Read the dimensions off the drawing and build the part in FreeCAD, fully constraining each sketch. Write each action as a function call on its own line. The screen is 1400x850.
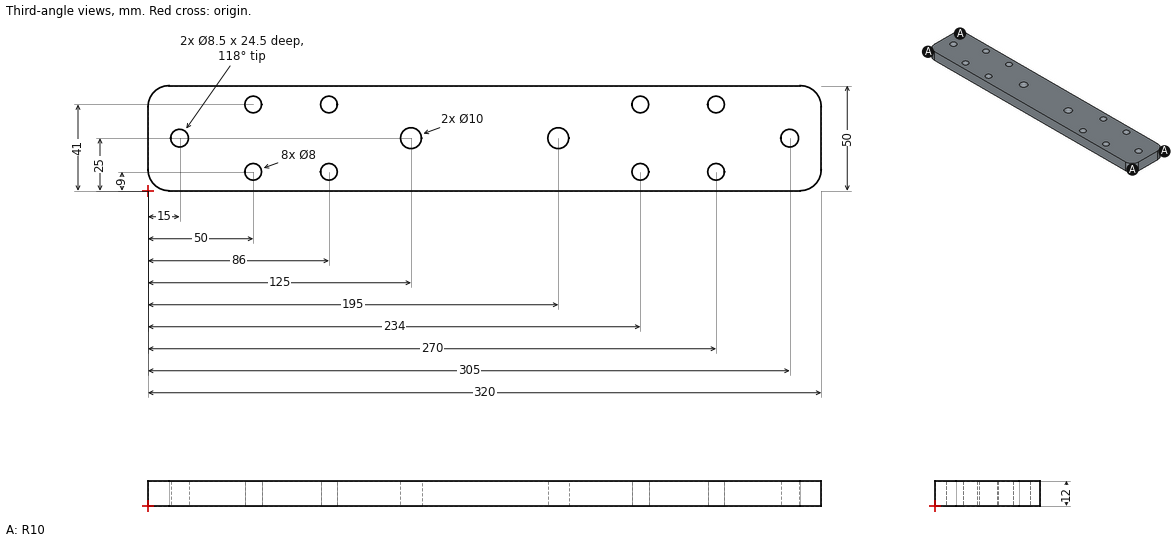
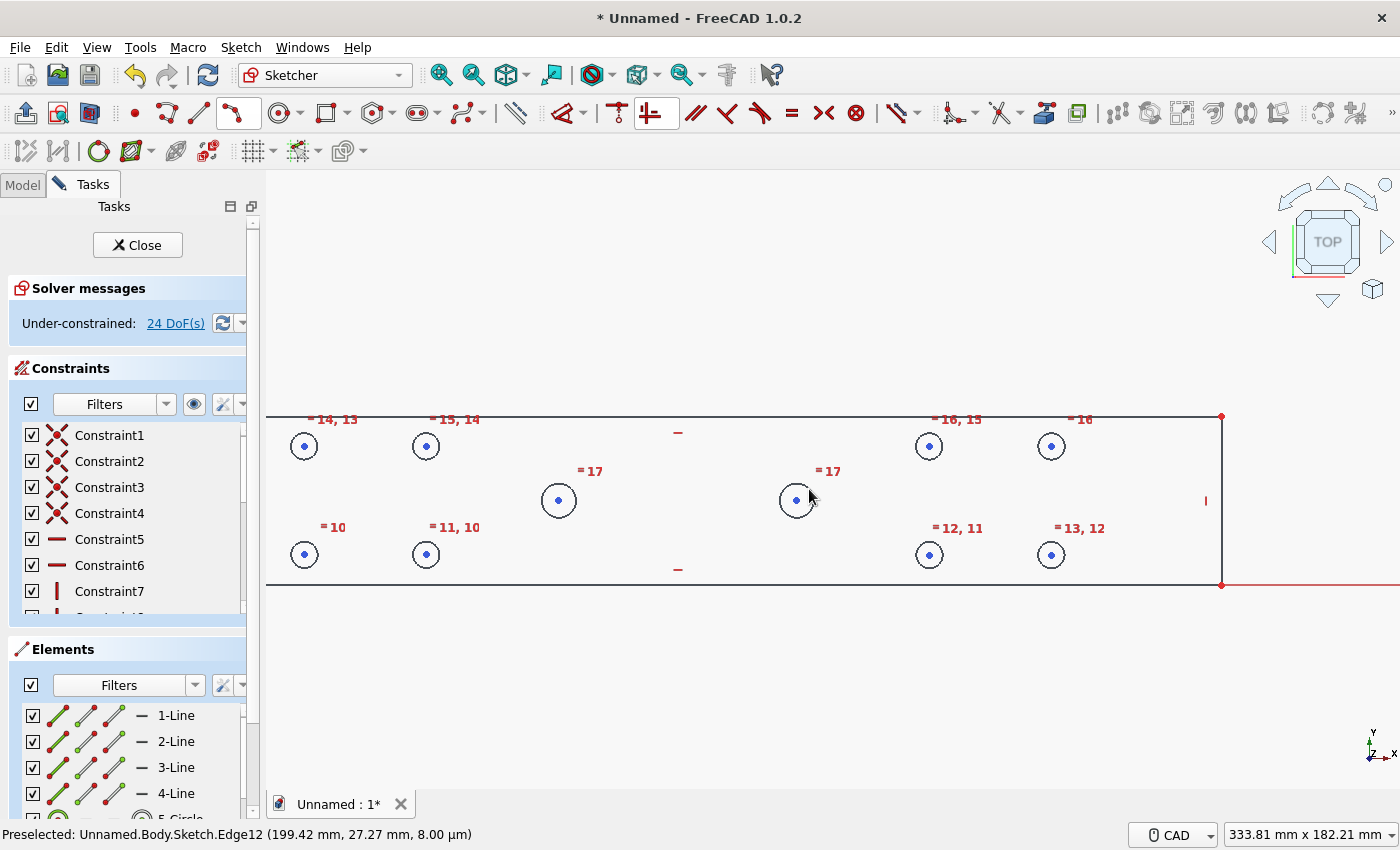
scroll(314, 545, up, 2)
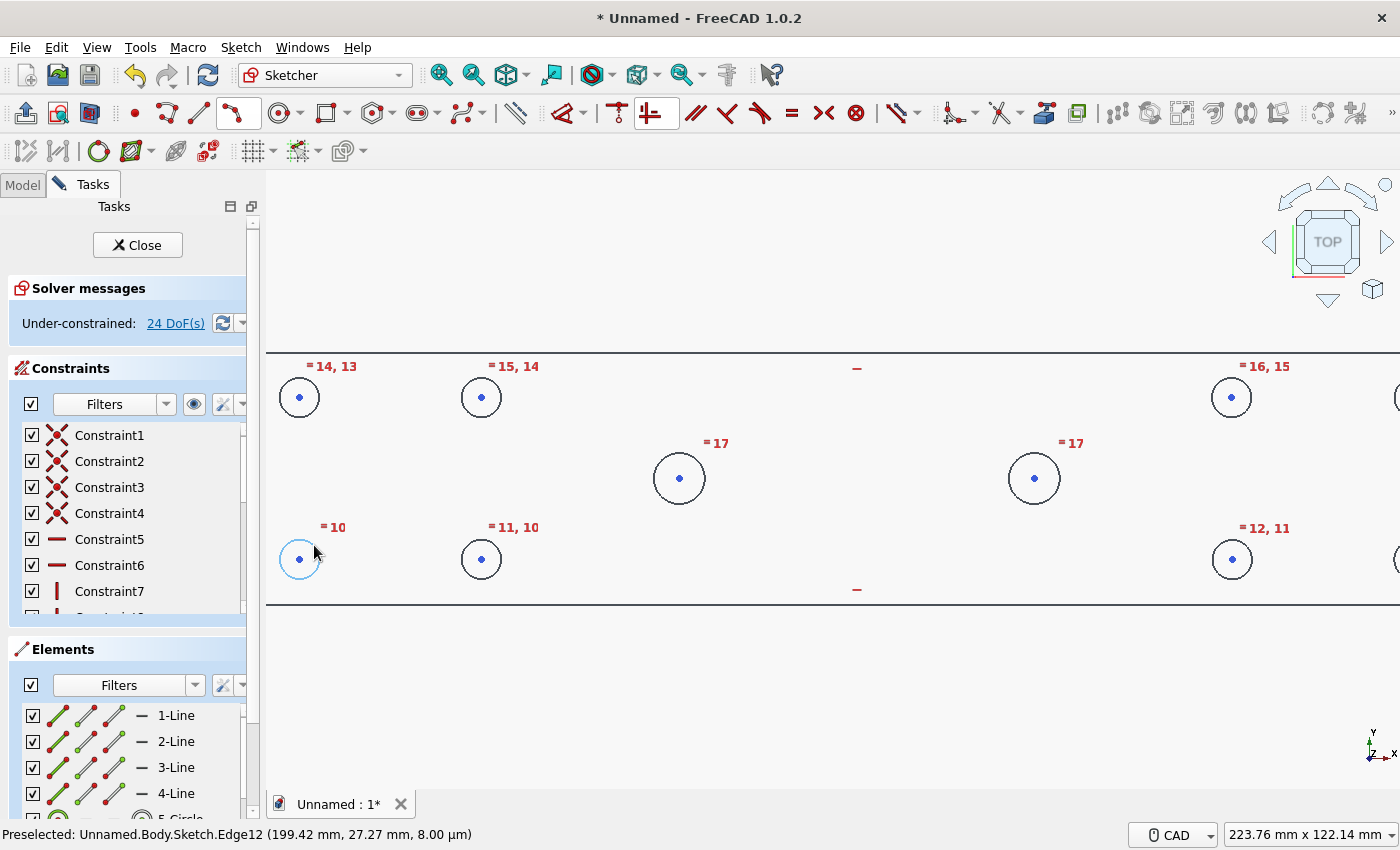
click(314, 545)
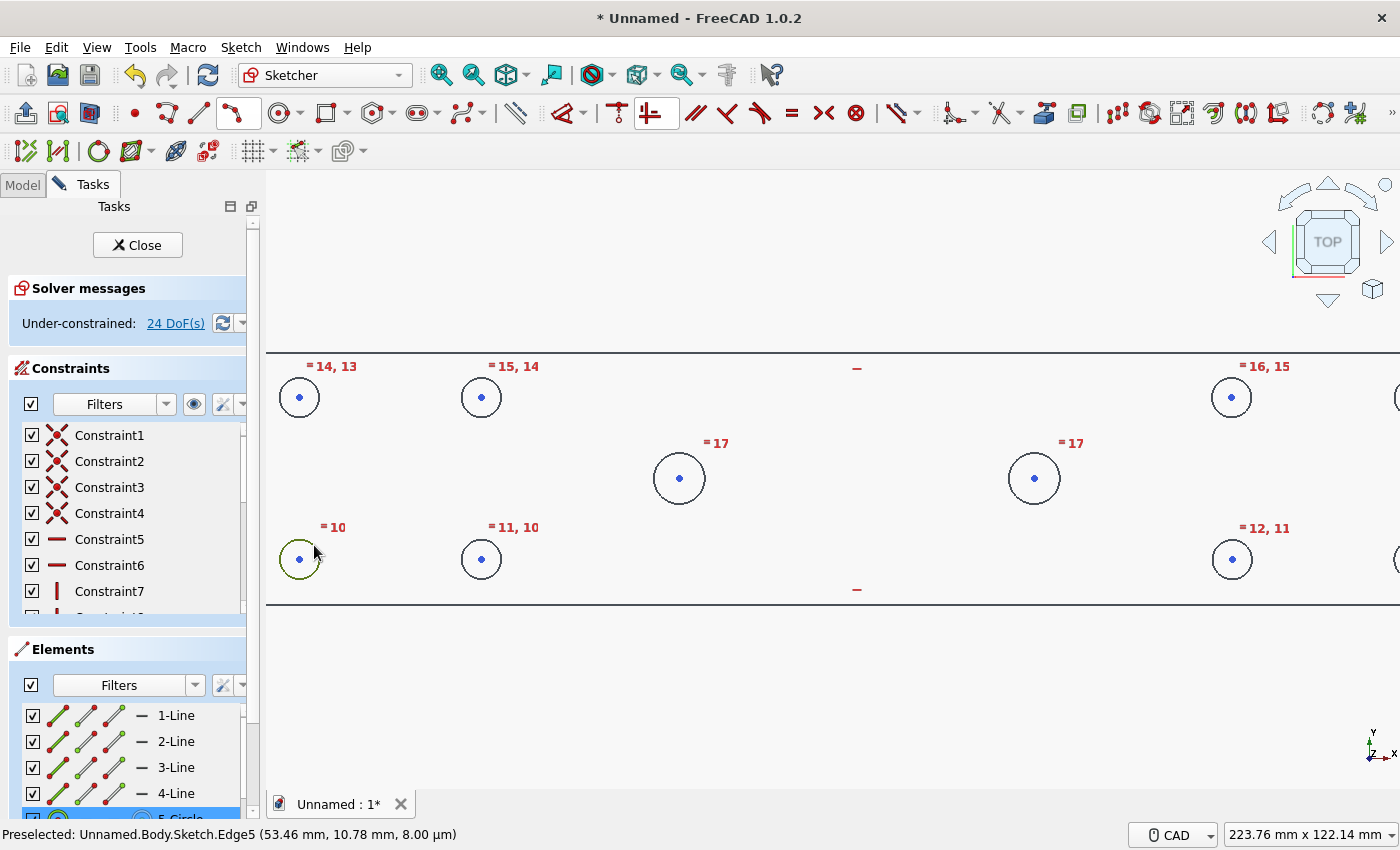
key(k)
key(o)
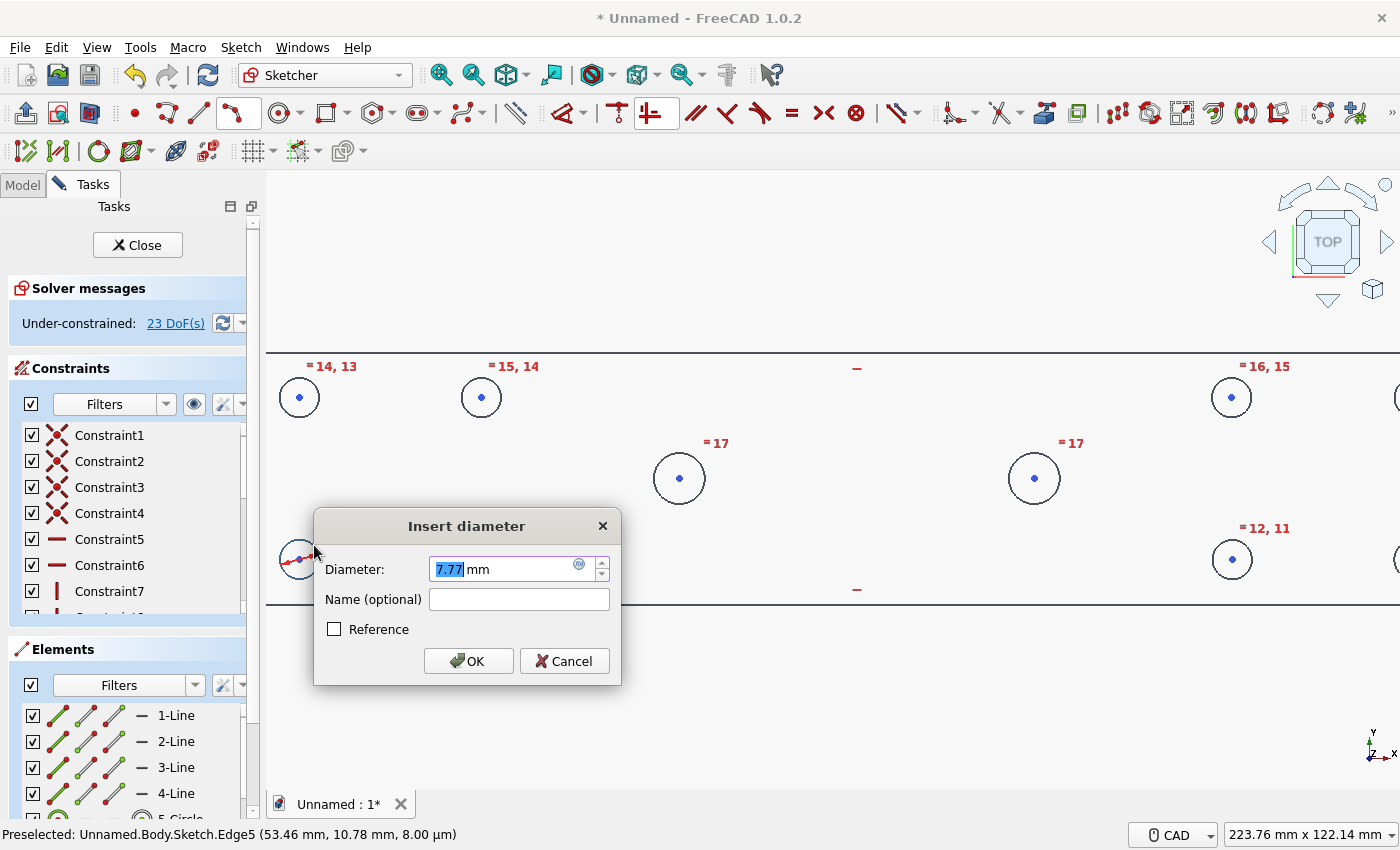
text(8)
key(Return)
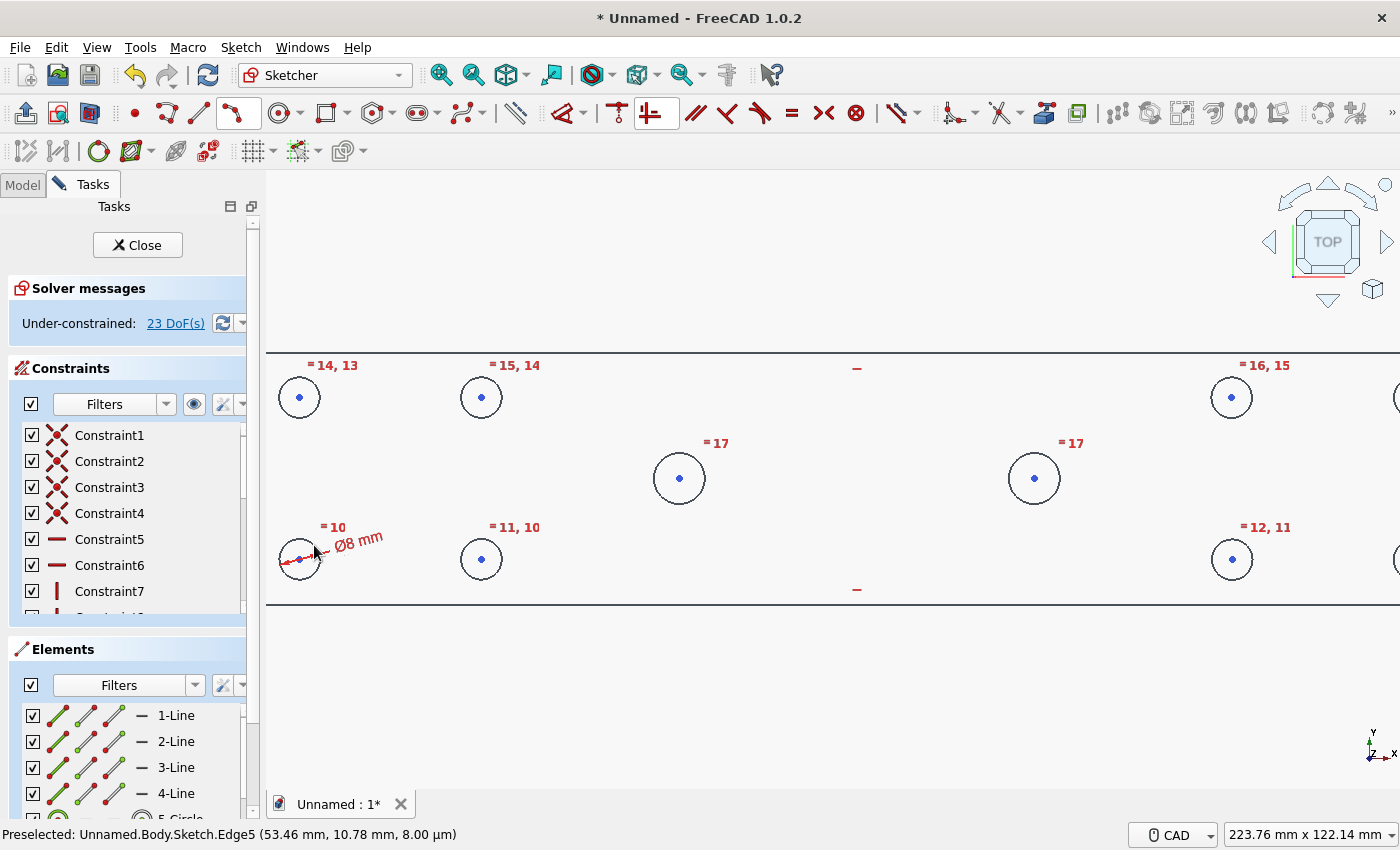
click(697, 461)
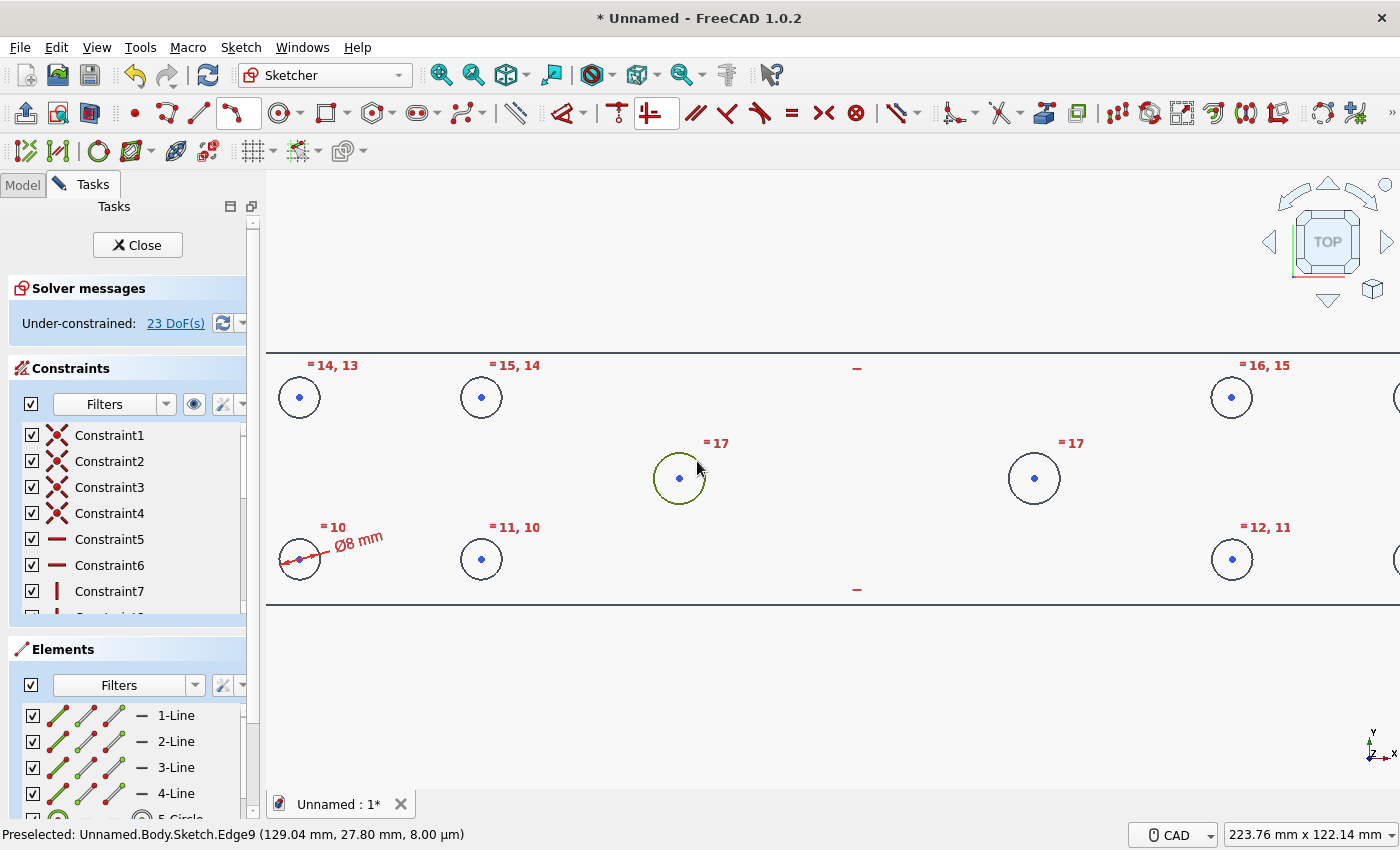
click(586, 114)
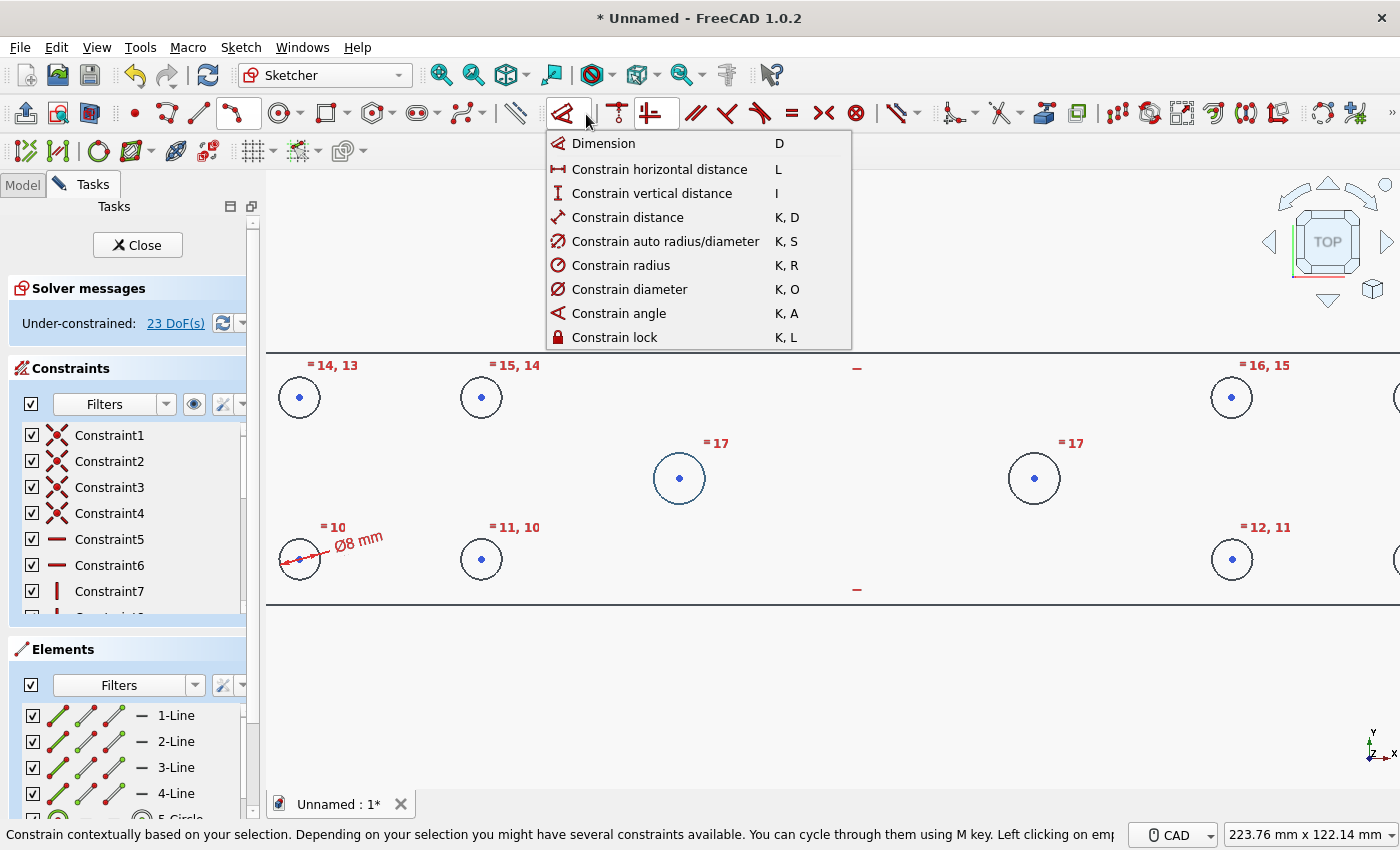
click(699, 289)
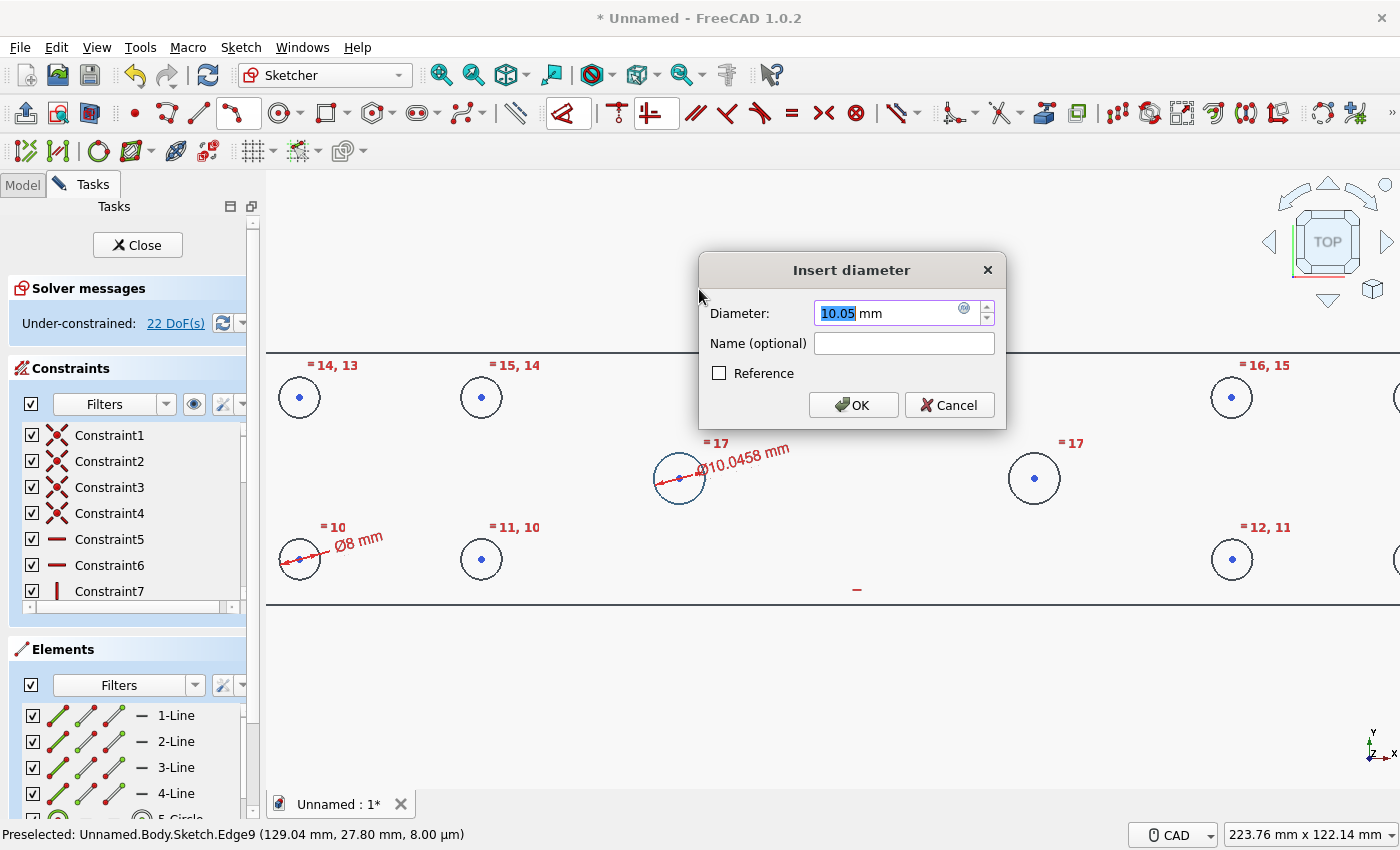
text(10)
key(Return)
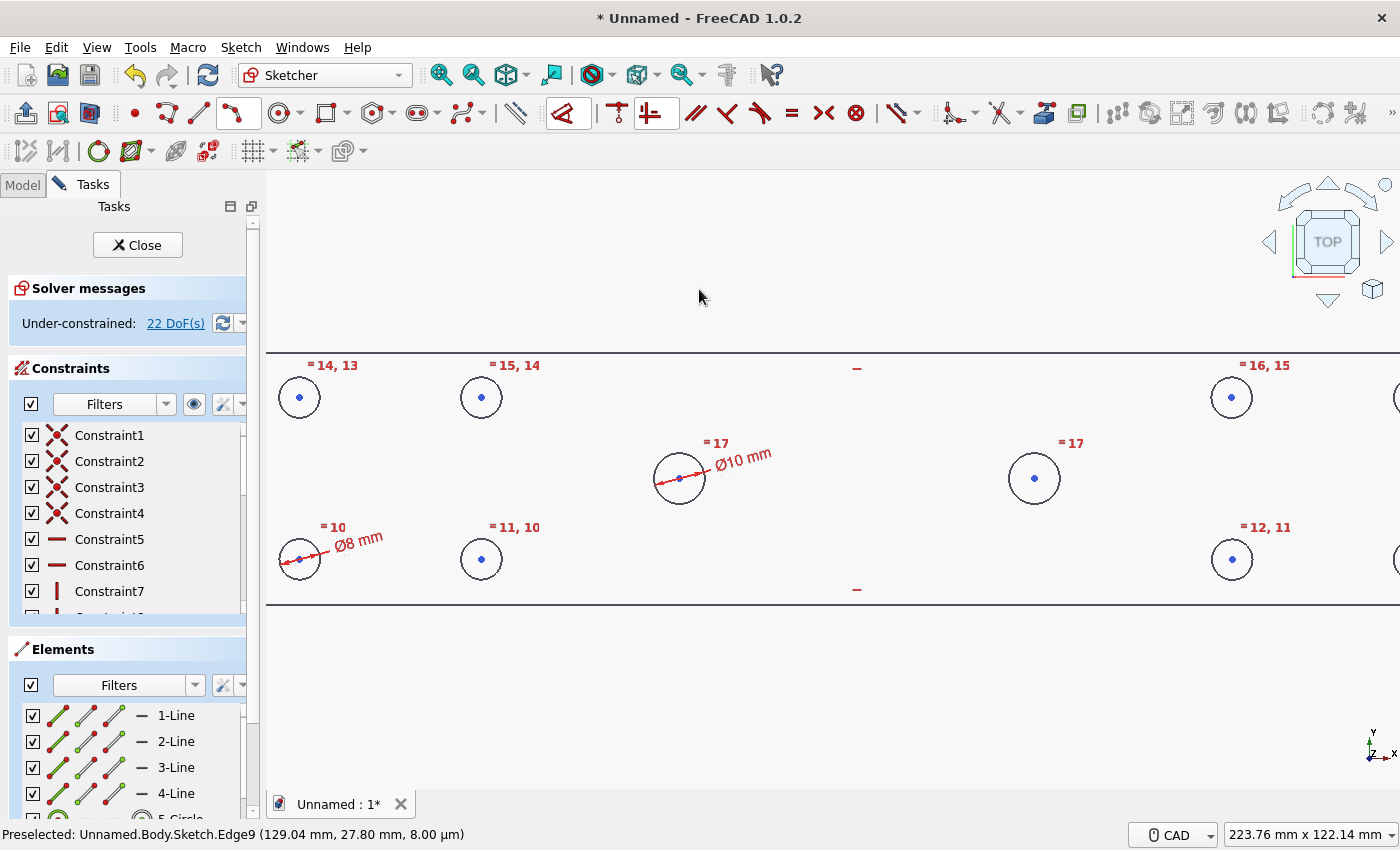
click(300, 559)